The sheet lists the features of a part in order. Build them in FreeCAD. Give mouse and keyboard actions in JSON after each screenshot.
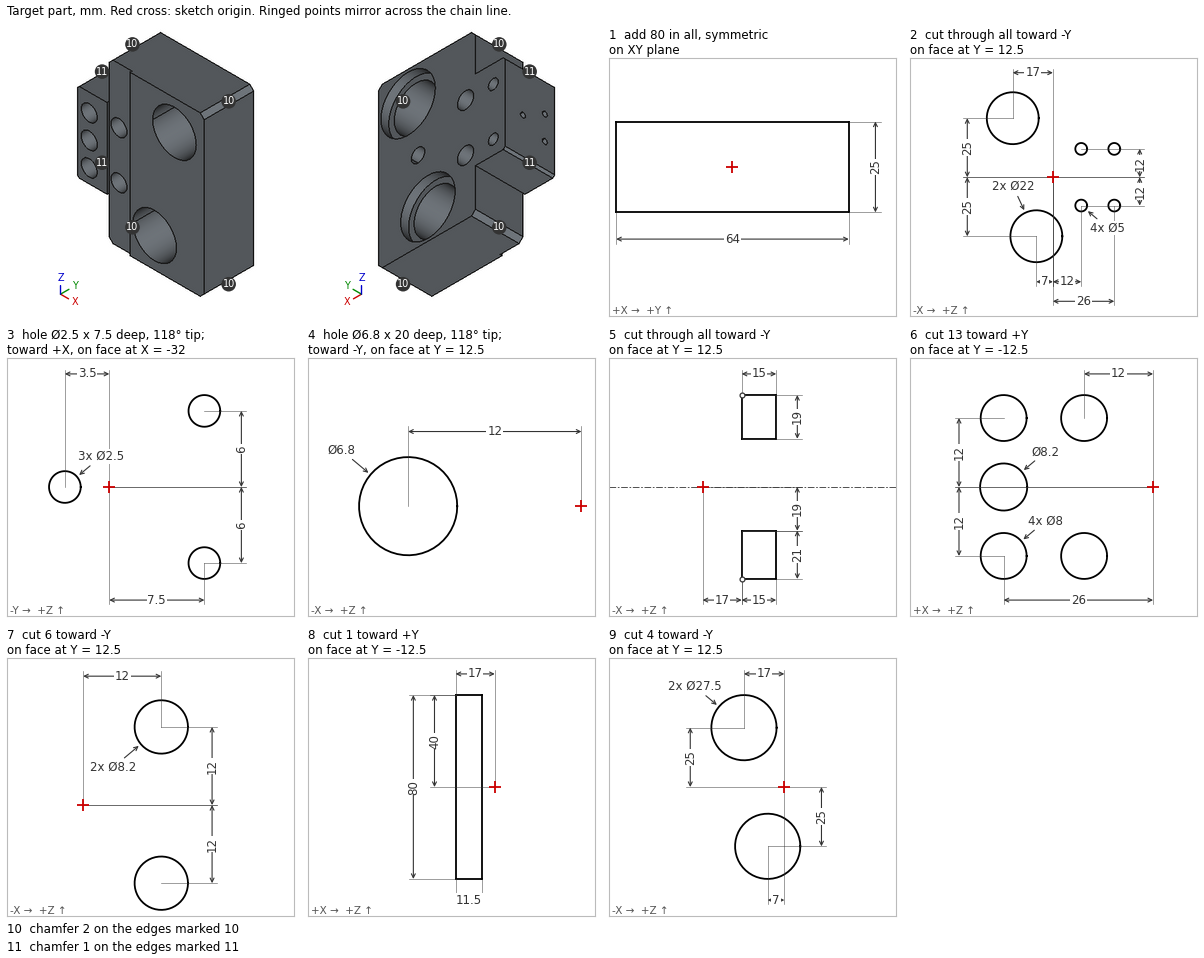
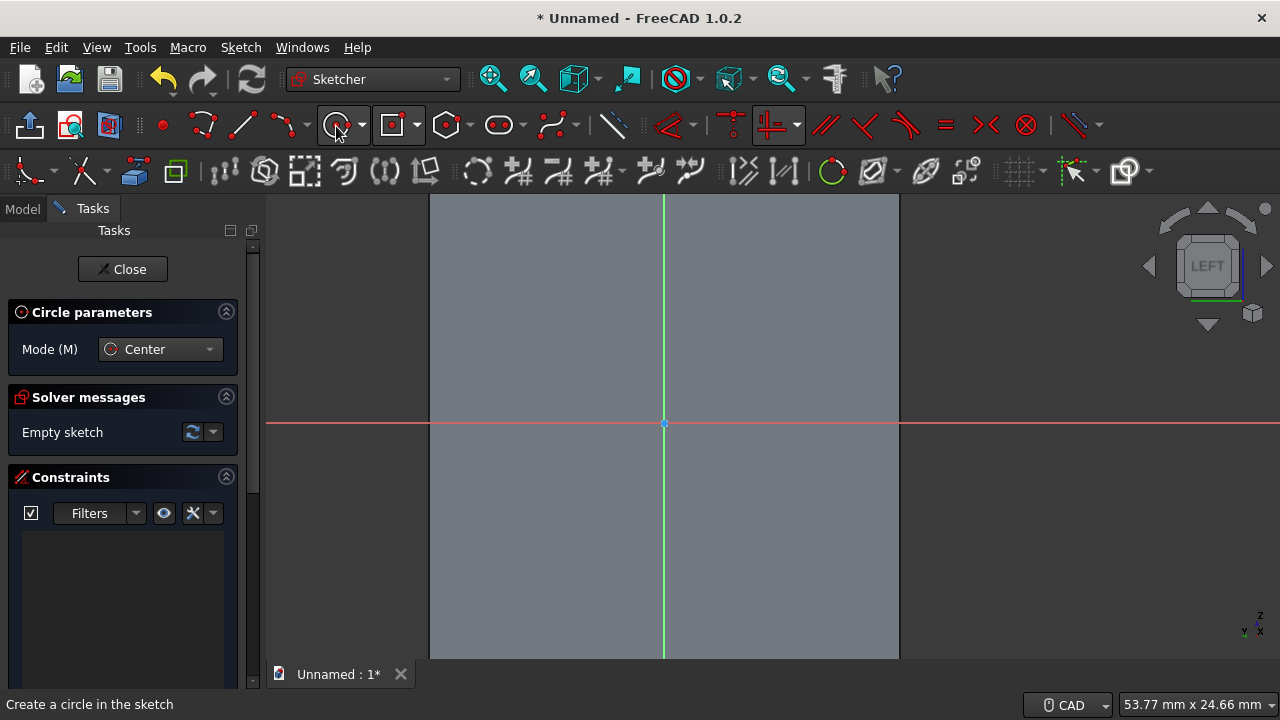
{"action": "left_click", "coordinate": [598, 423]}
{"action": "left_click", "coordinate": [615, 407]}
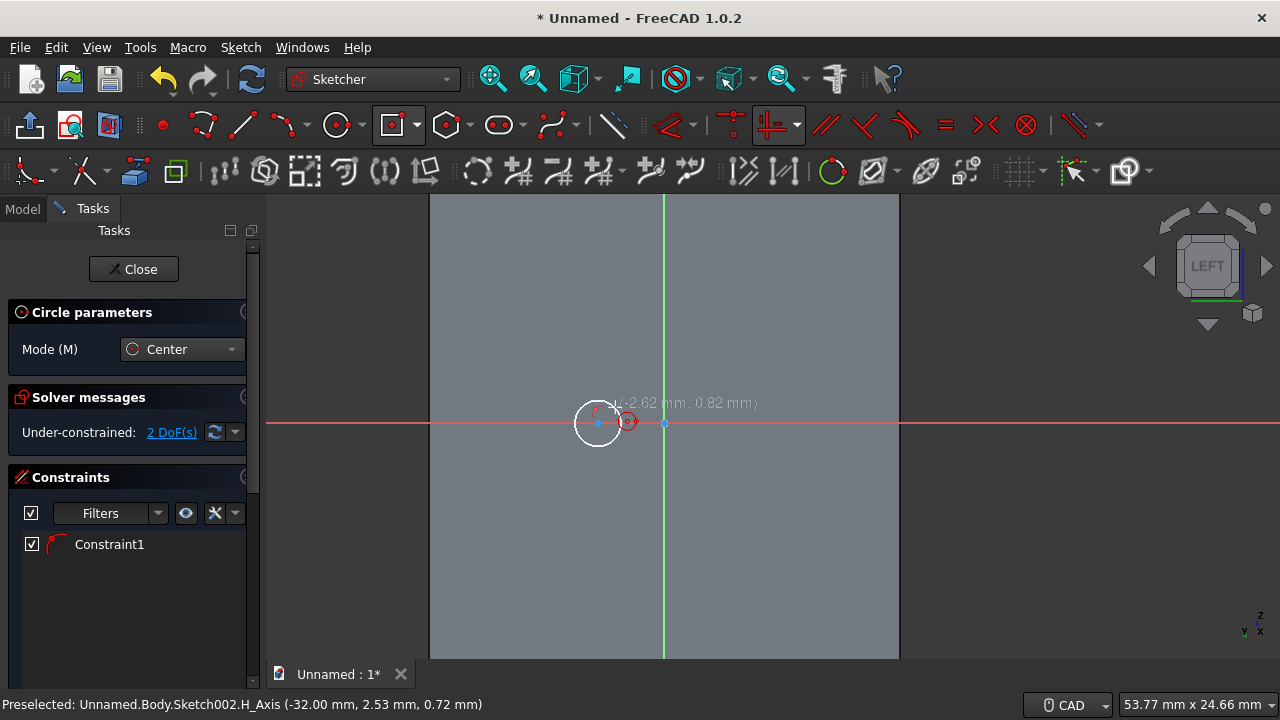
{"action": "left_click", "coordinate": [806, 537]}
{"action": "left_click", "coordinate": [823, 520]}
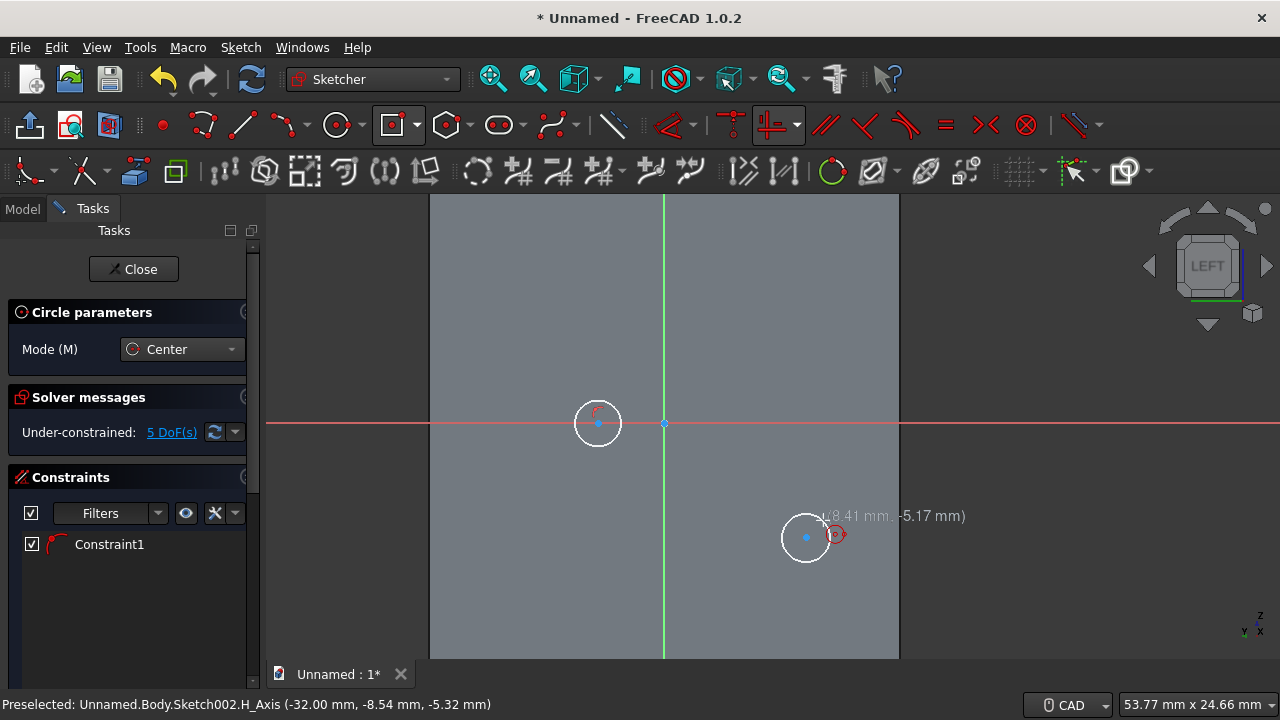
{"action": "left_click", "coordinate": [806, 310]}
{"action": "left_click", "coordinate": [823, 294]}
{"action": "key", "text": "Escape"}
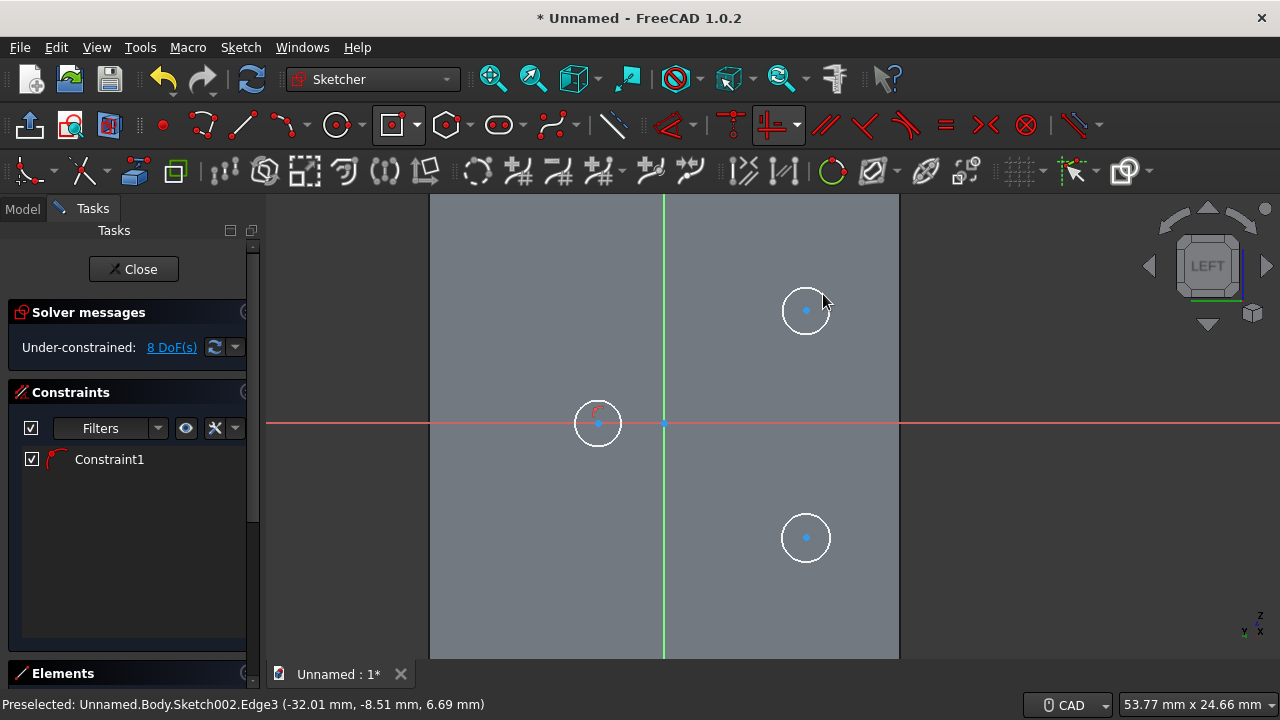
{"action": "left_click", "coordinate": [614, 407]}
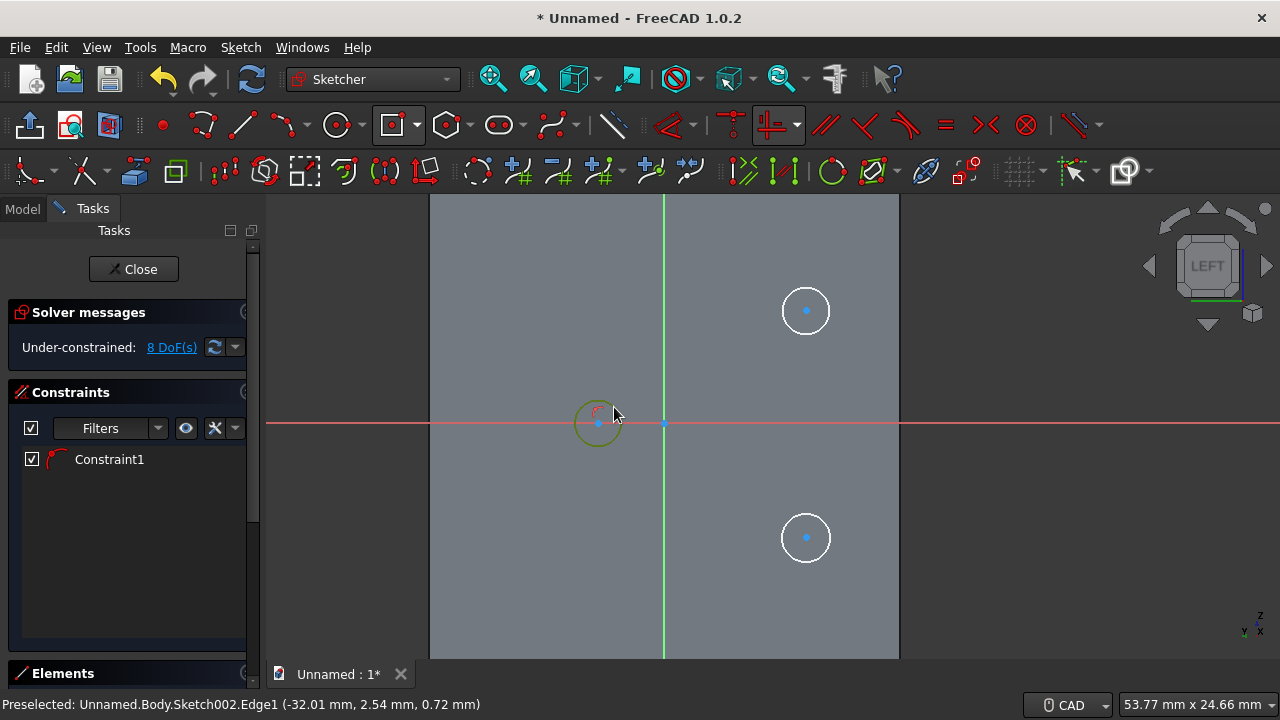
{"action": "left_click", "coordinate": [823, 521]}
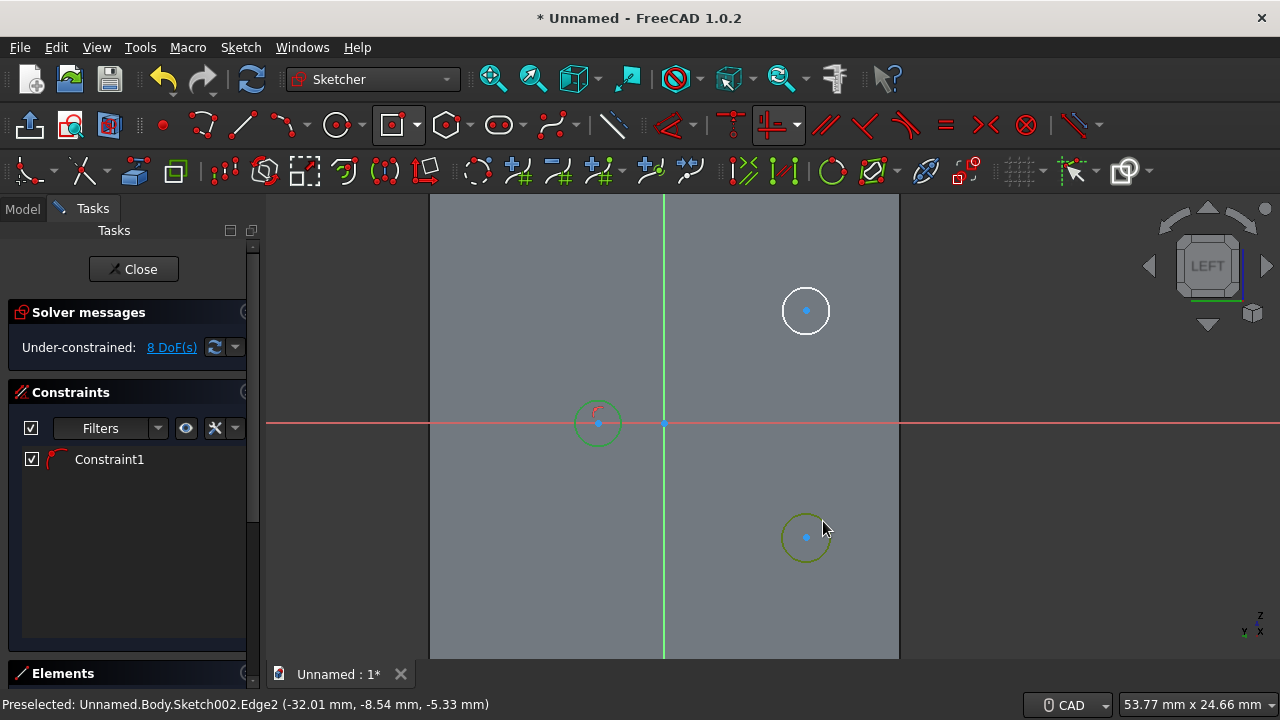
{"action": "left_click", "coordinate": [822, 294]}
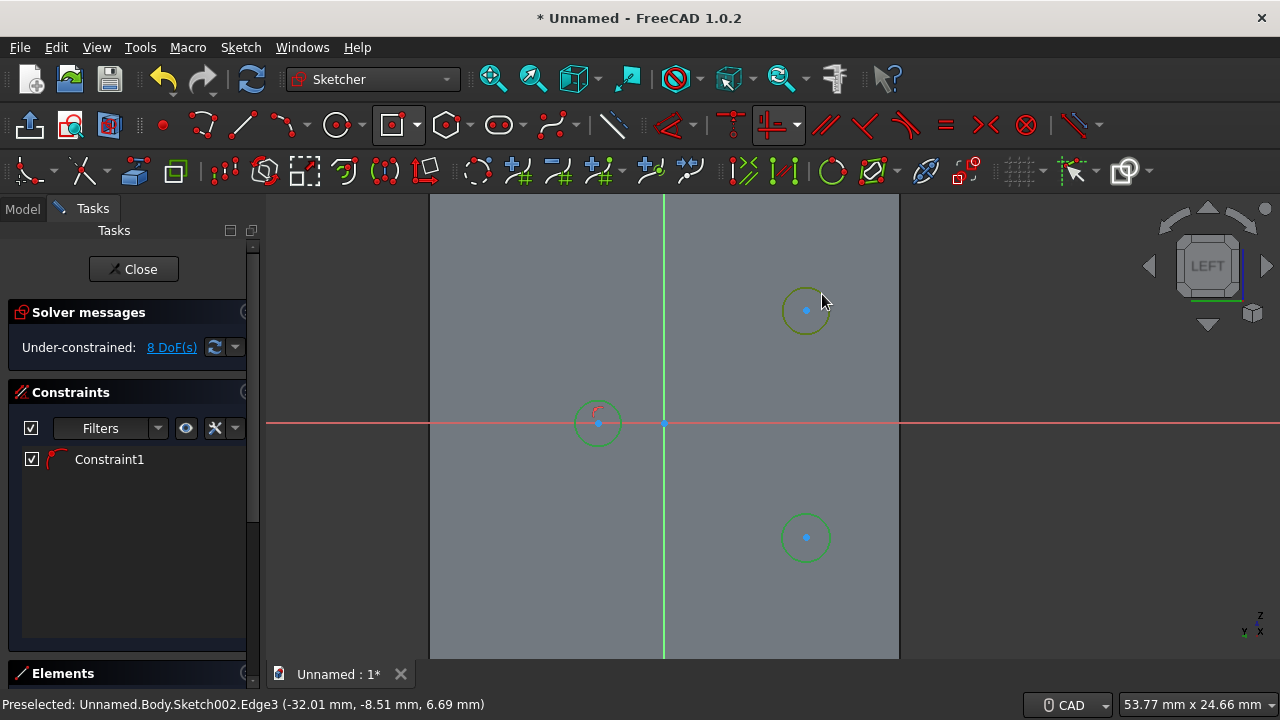
{"action": "left_click", "coordinate": [946, 126]}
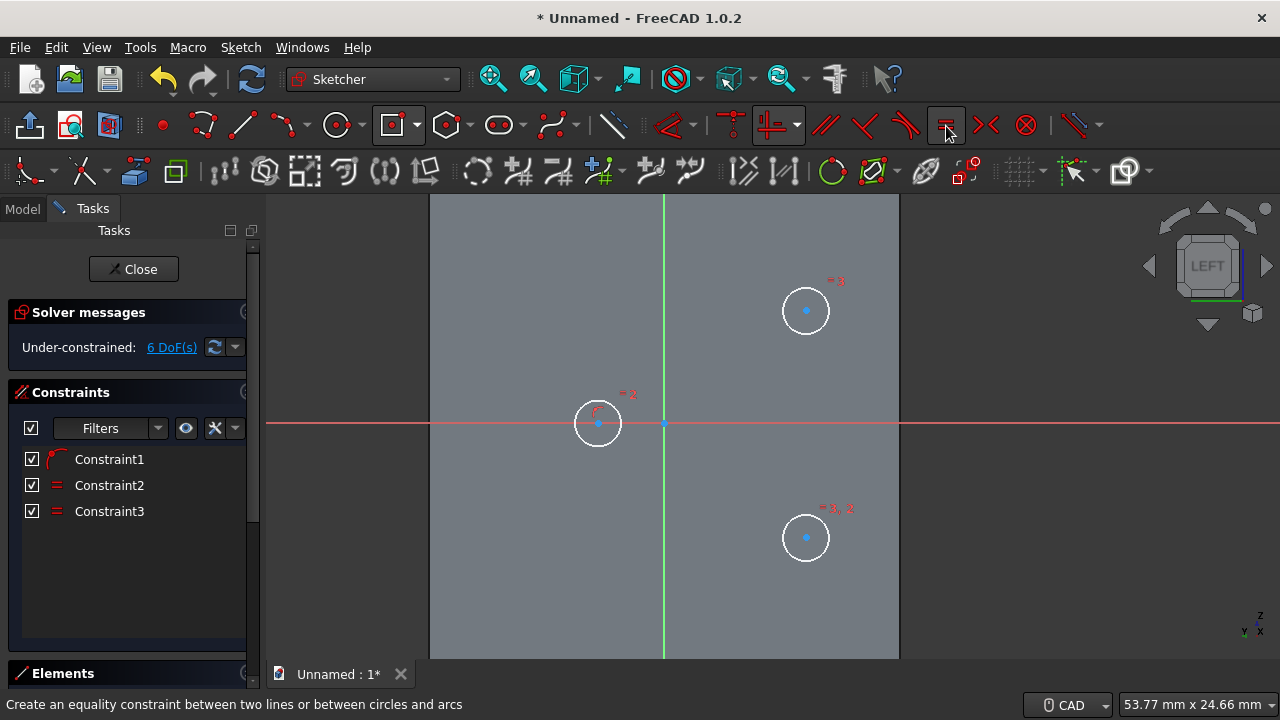
{"action": "left_click", "coordinate": [806, 538]}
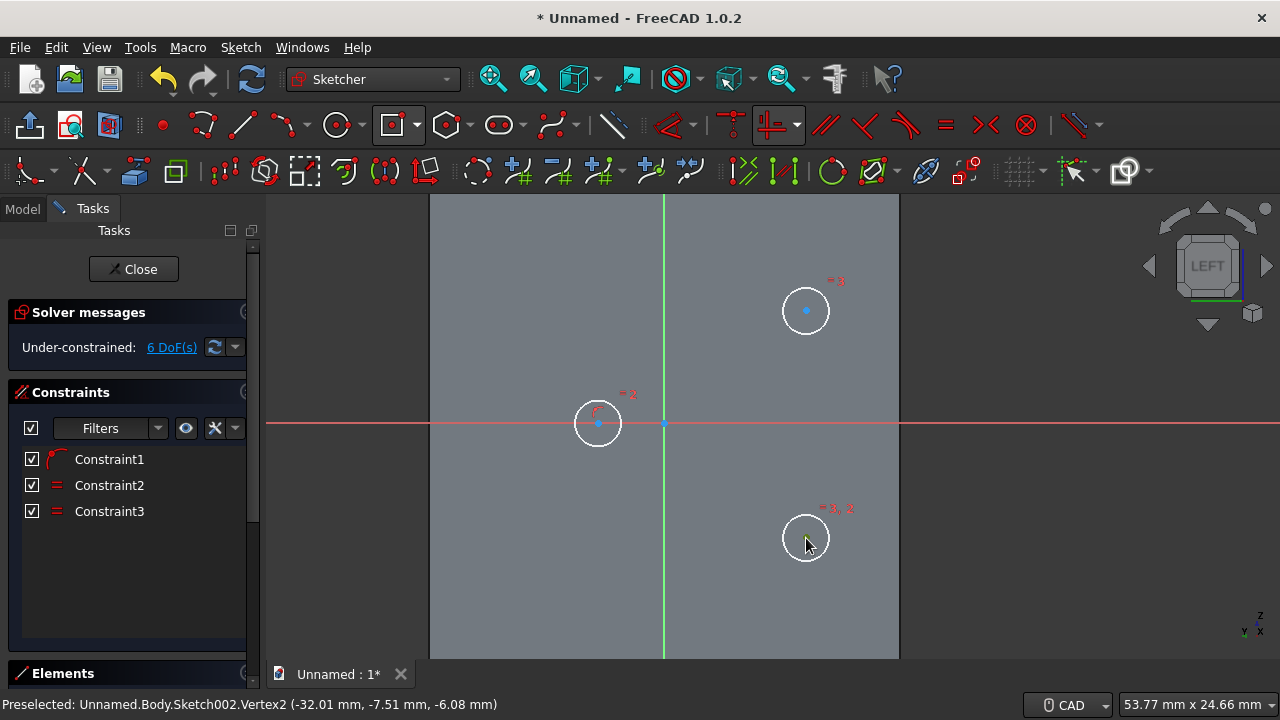
{"action": "left_click", "coordinate": [806, 311]}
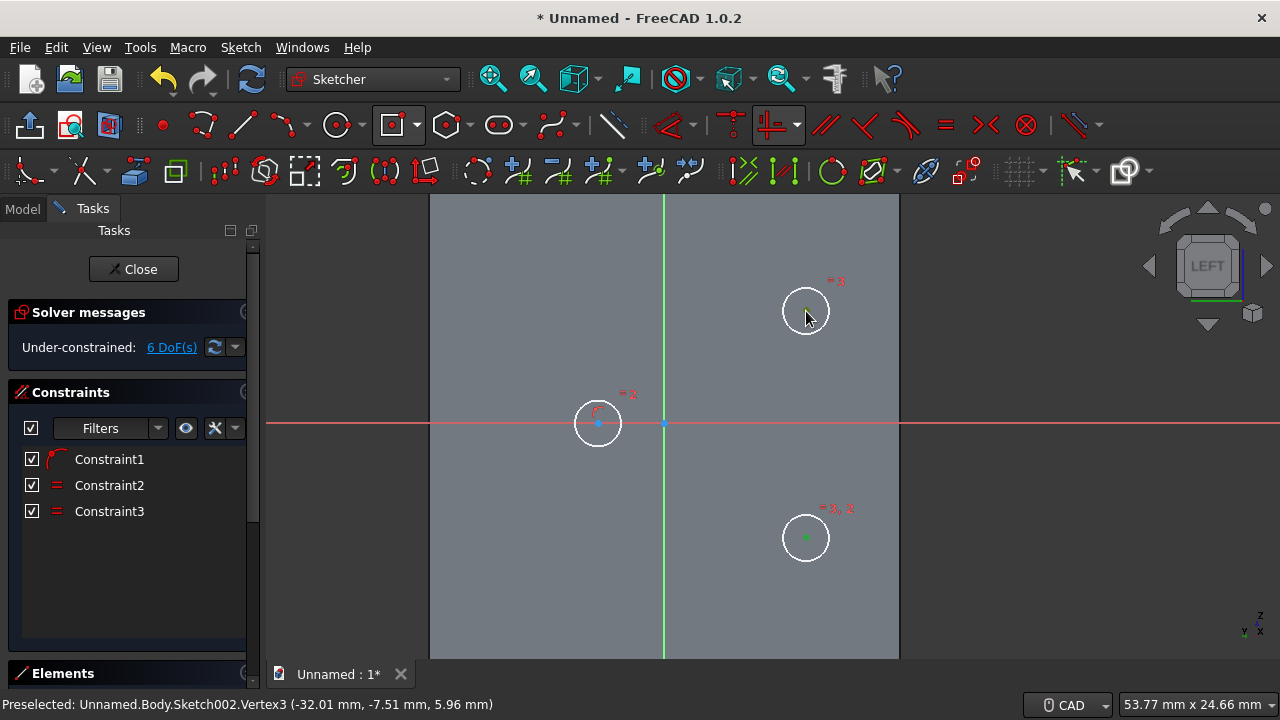
{"action": "key", "text": "v"}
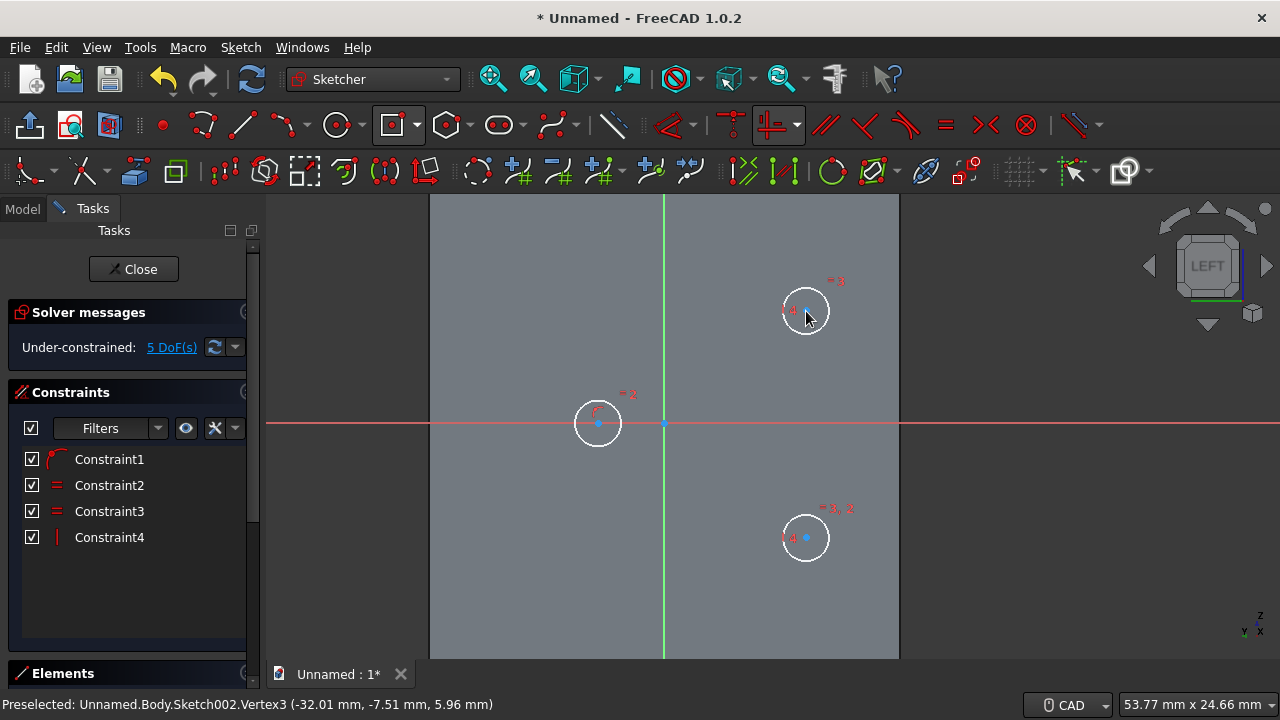
{"action": "left_click", "coordinate": [668, 126]}